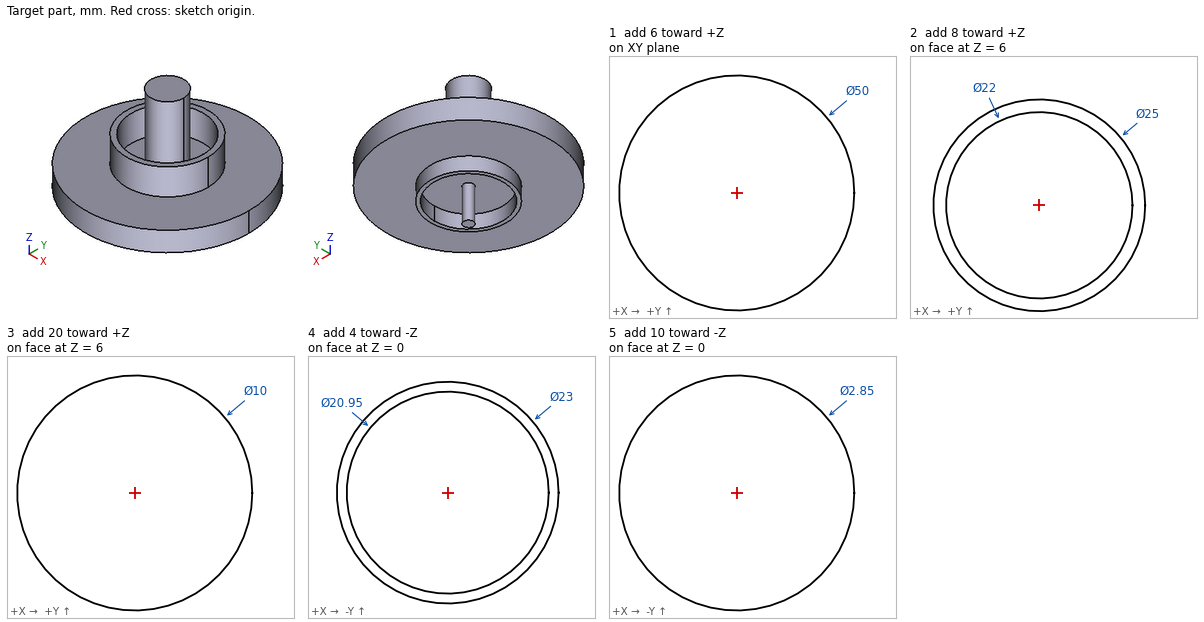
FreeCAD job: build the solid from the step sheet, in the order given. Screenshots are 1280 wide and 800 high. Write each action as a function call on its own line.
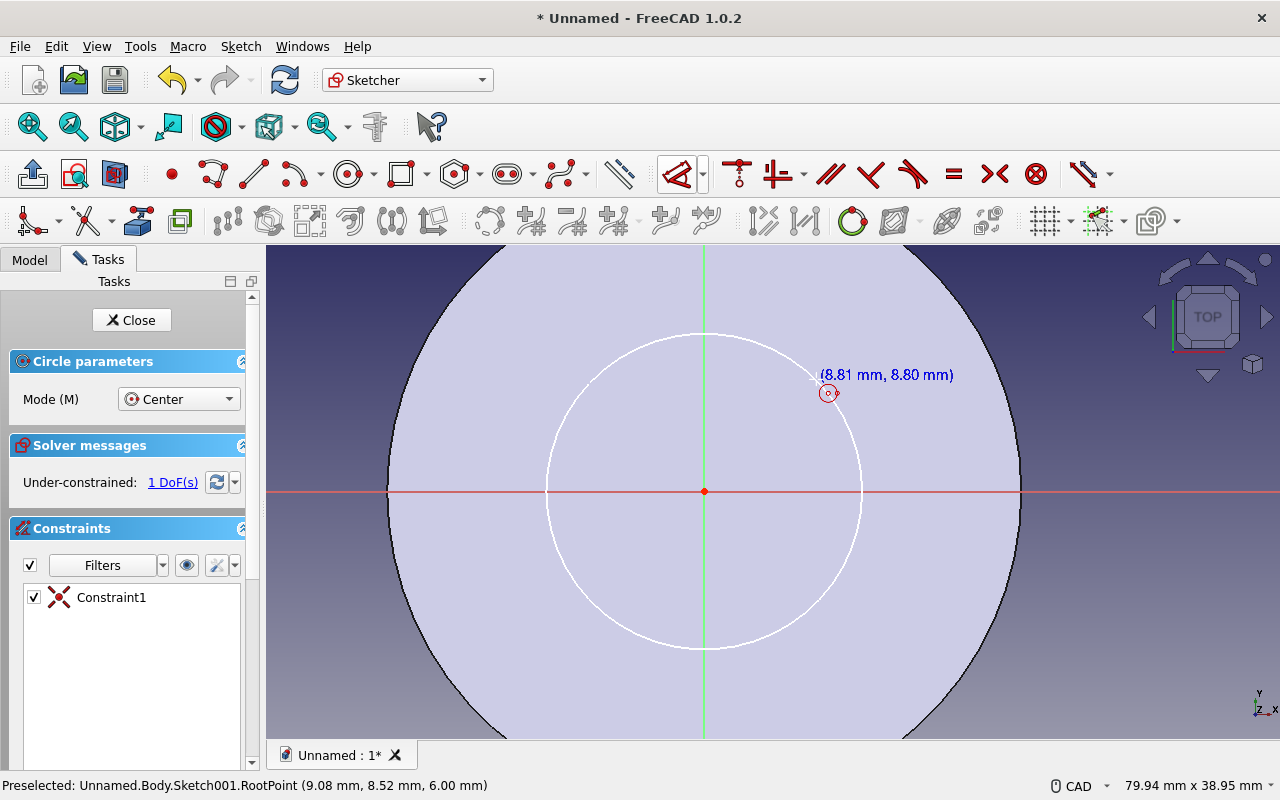
click(704, 492)
click(803, 393)
key(Escape)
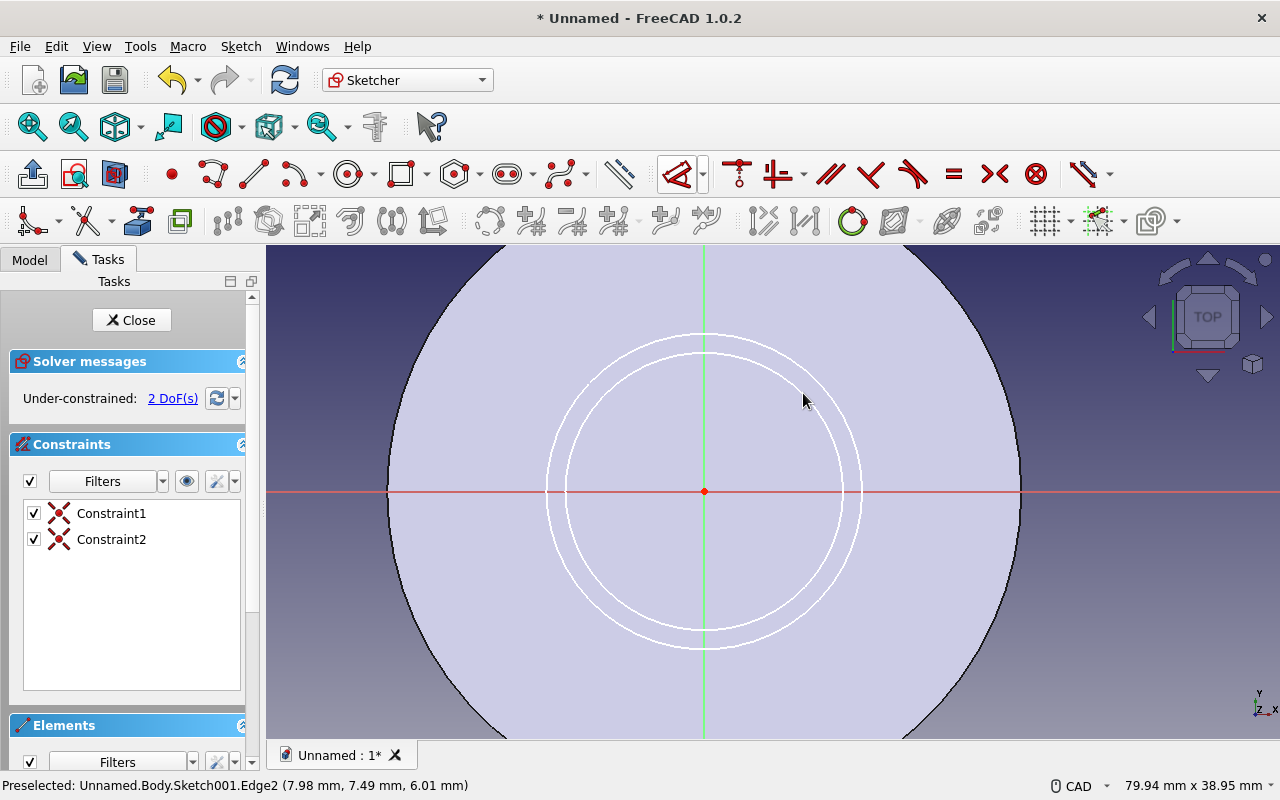
click(816, 380)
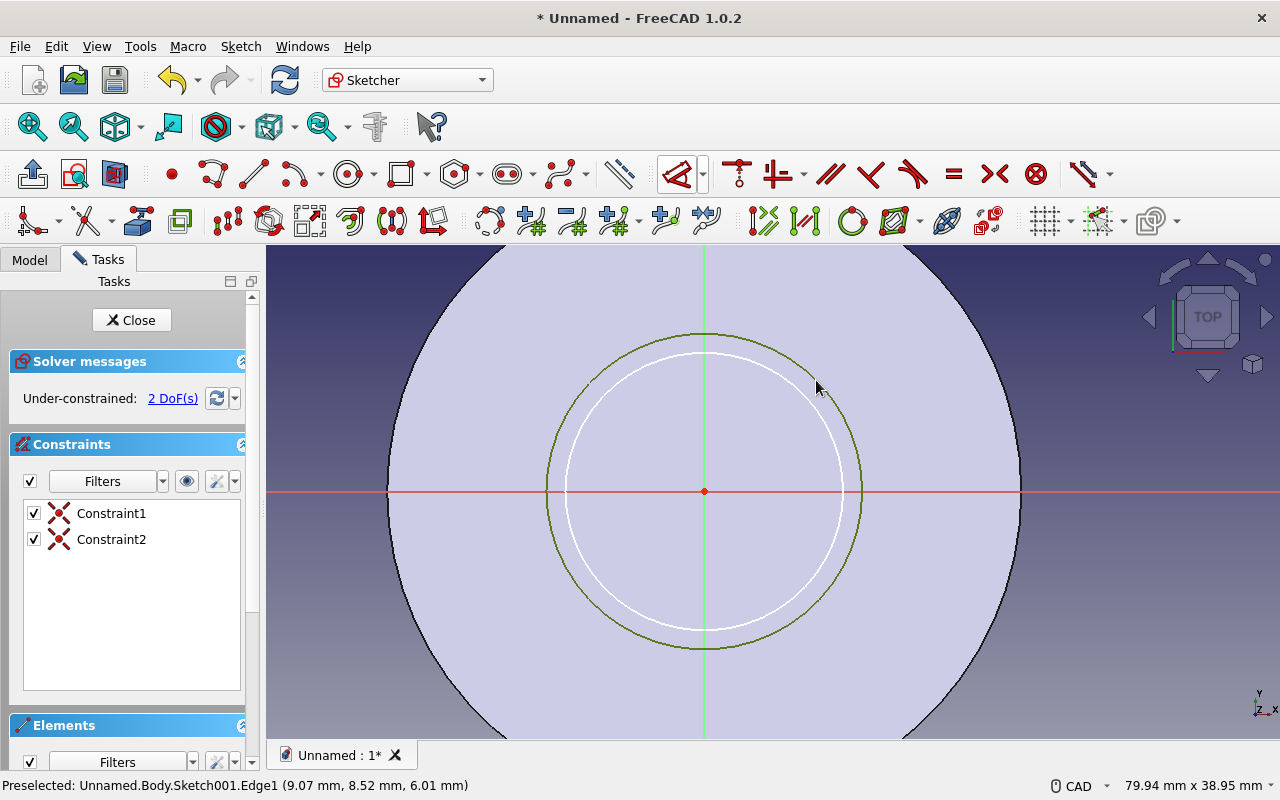
key(k)
key(o)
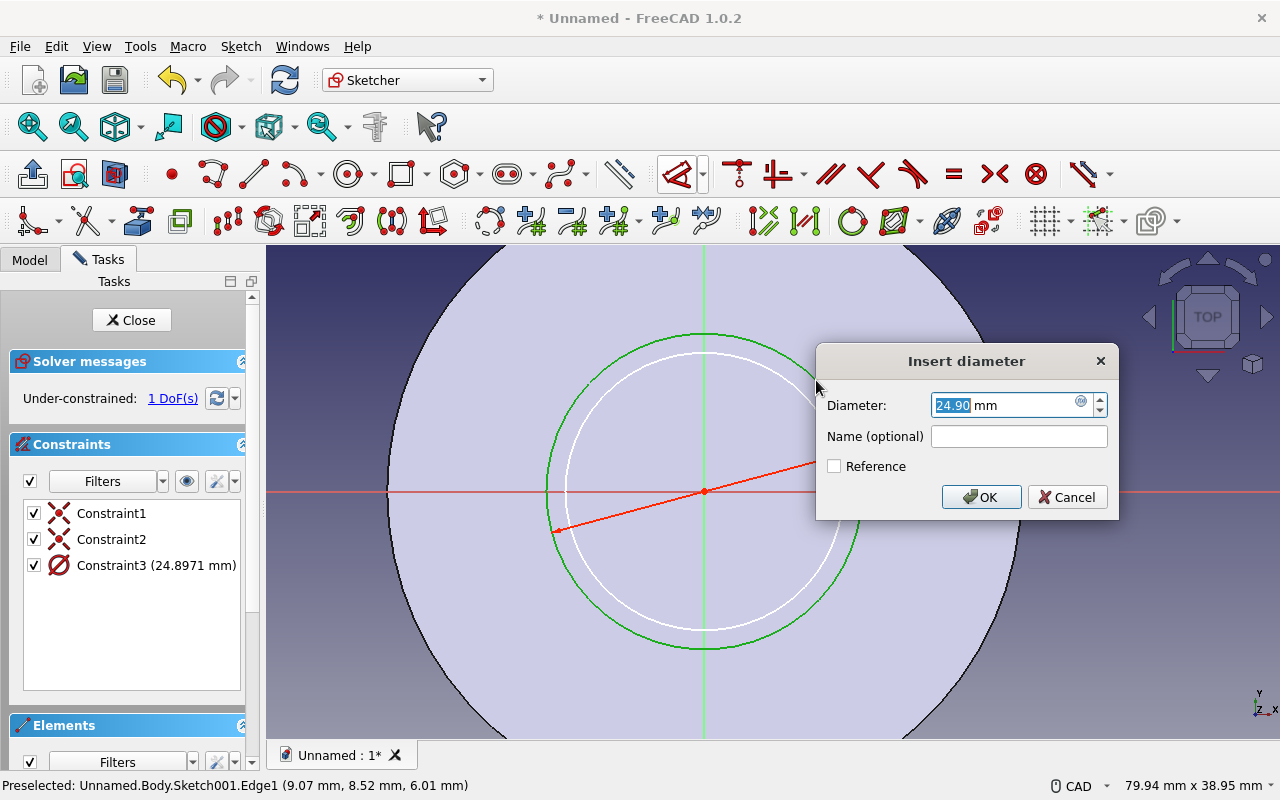
text(25)
key(Return)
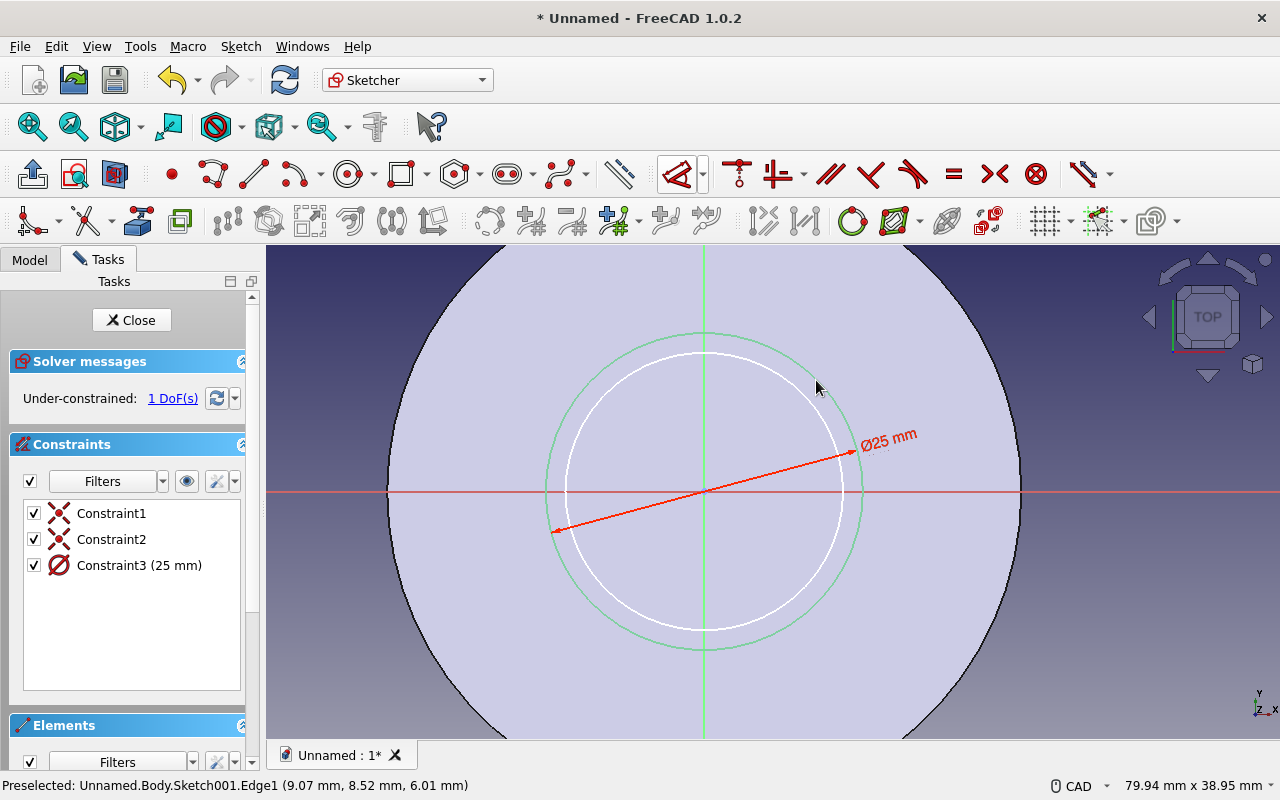
click(802, 393)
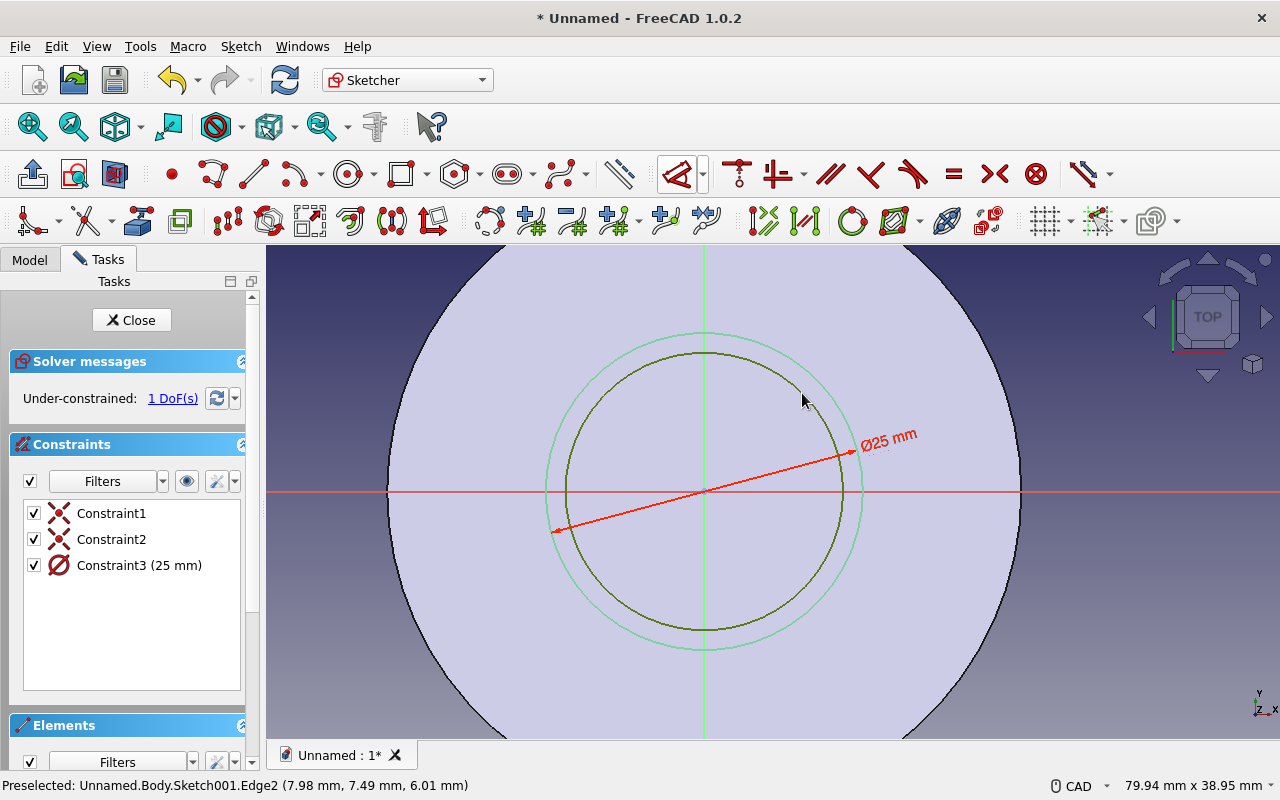
key(k)
key(o)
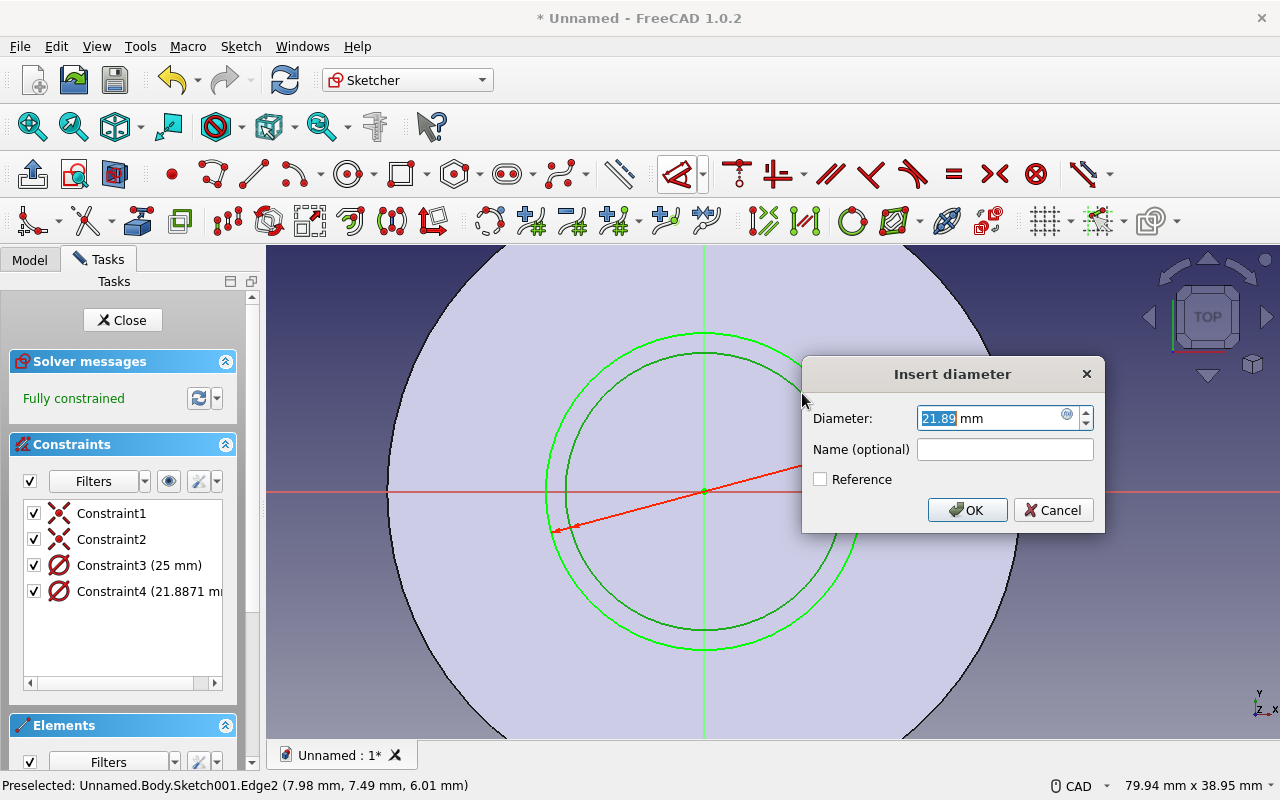
text(22)
key(Return)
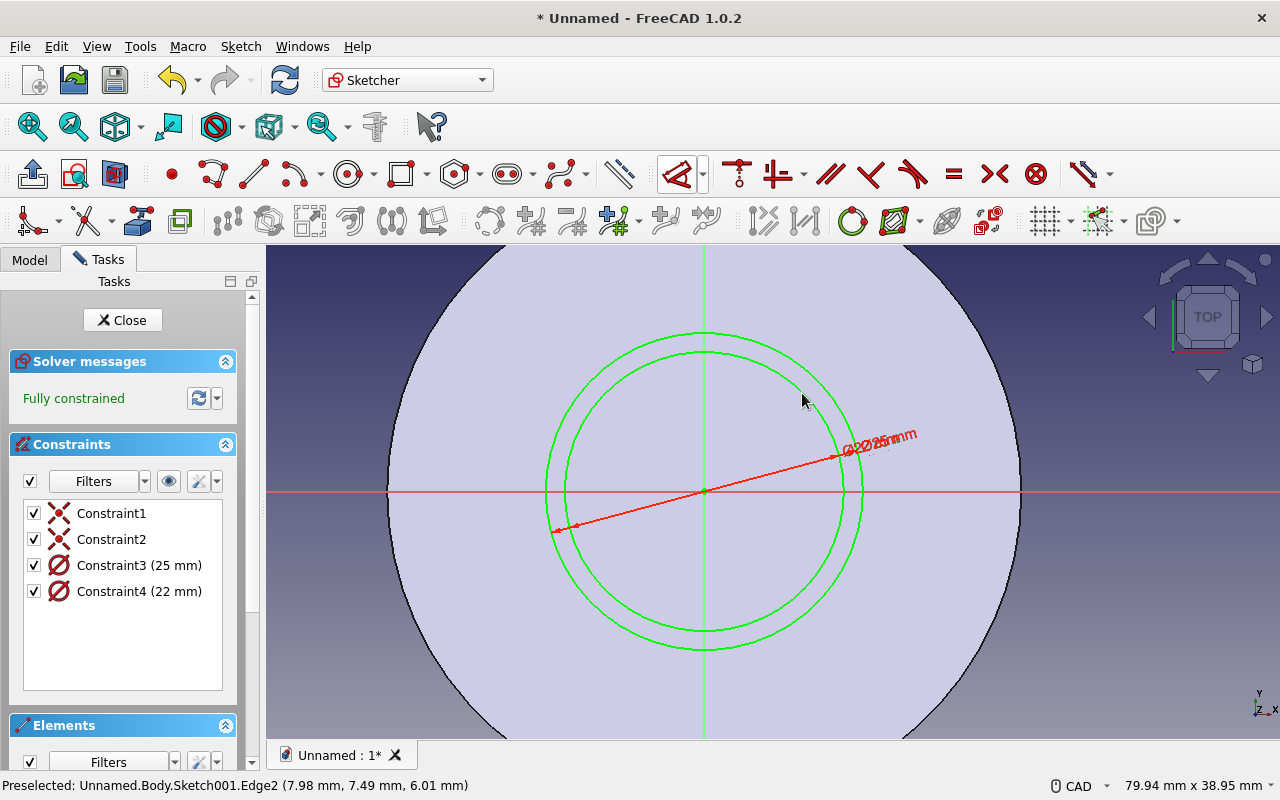
click(123, 320)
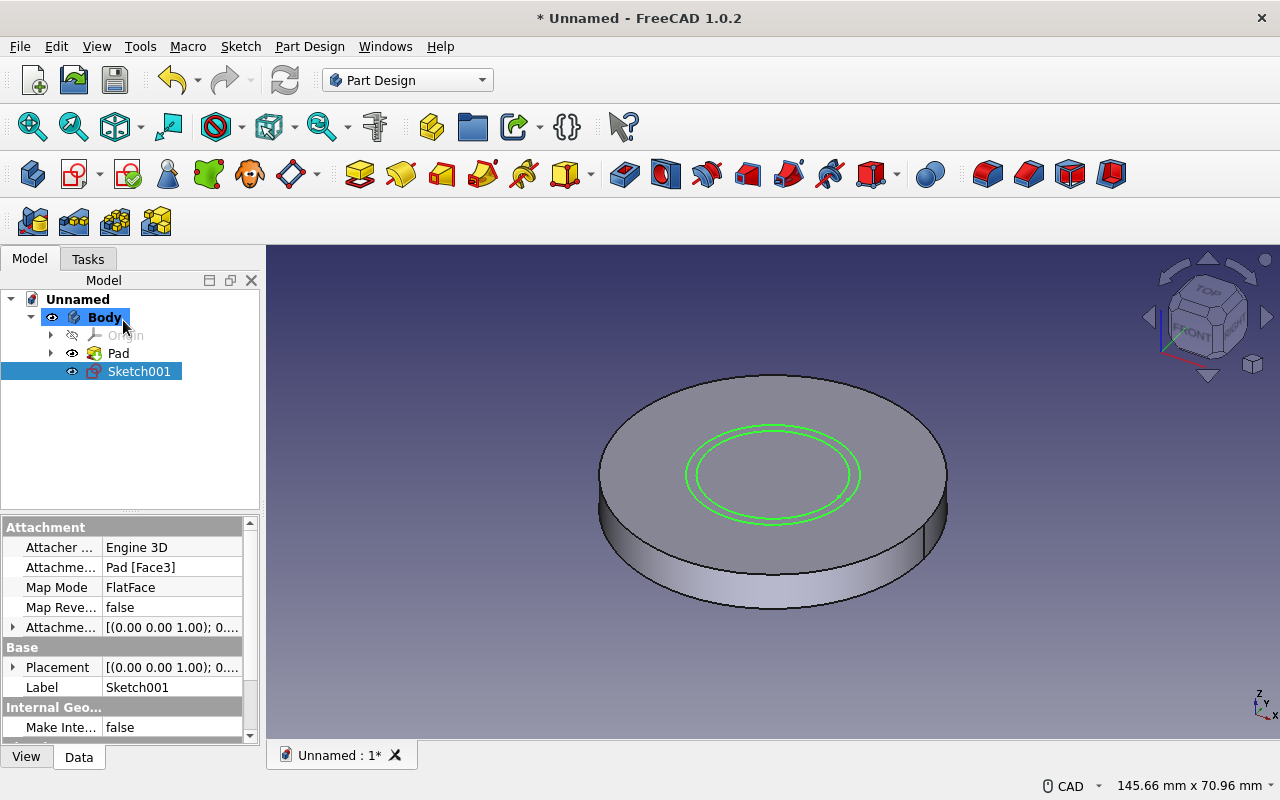
click(360, 174)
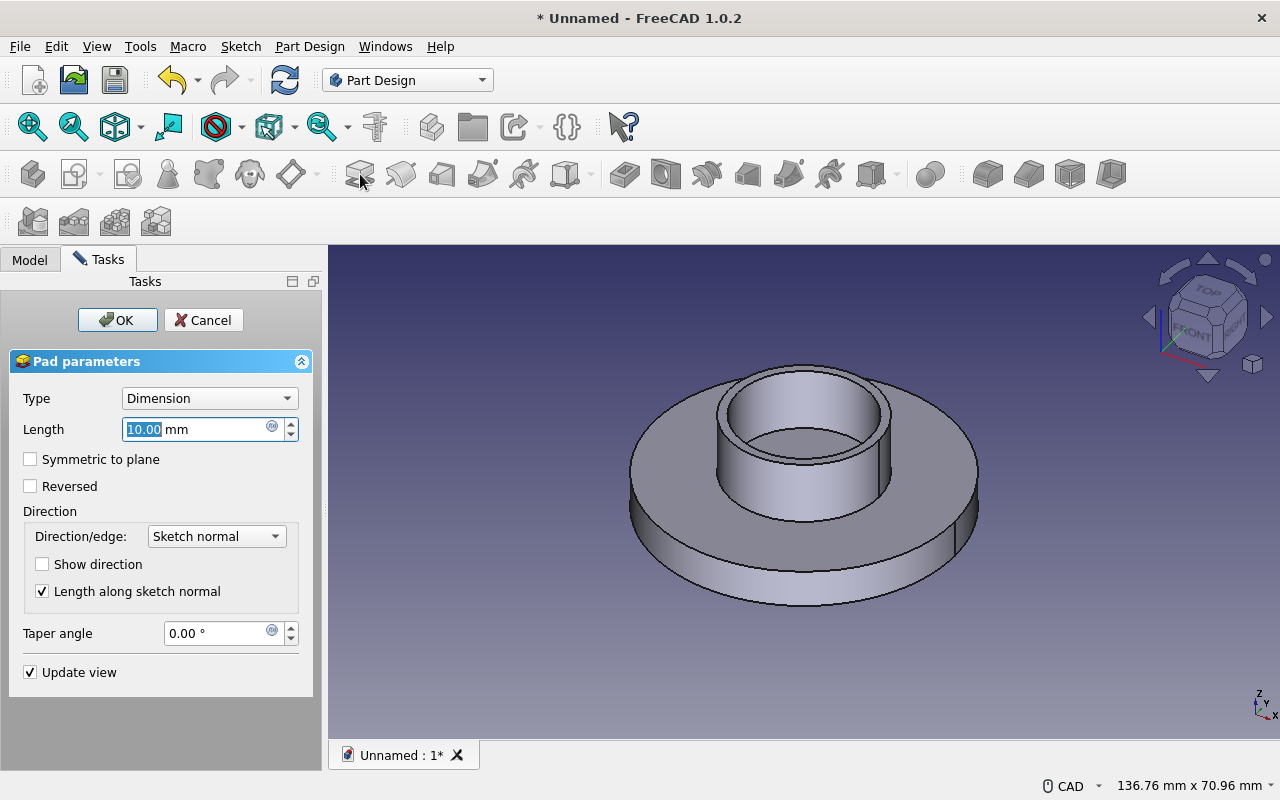
text(8)
key(Tab)